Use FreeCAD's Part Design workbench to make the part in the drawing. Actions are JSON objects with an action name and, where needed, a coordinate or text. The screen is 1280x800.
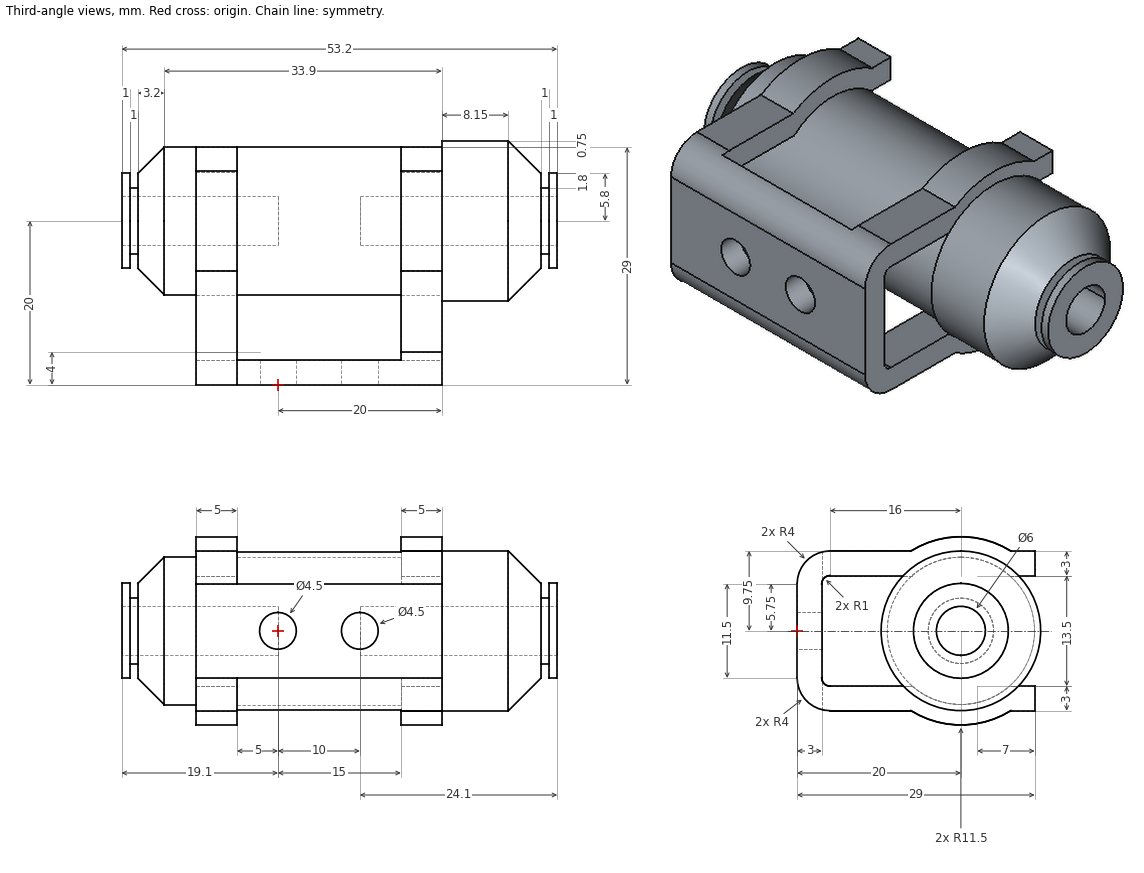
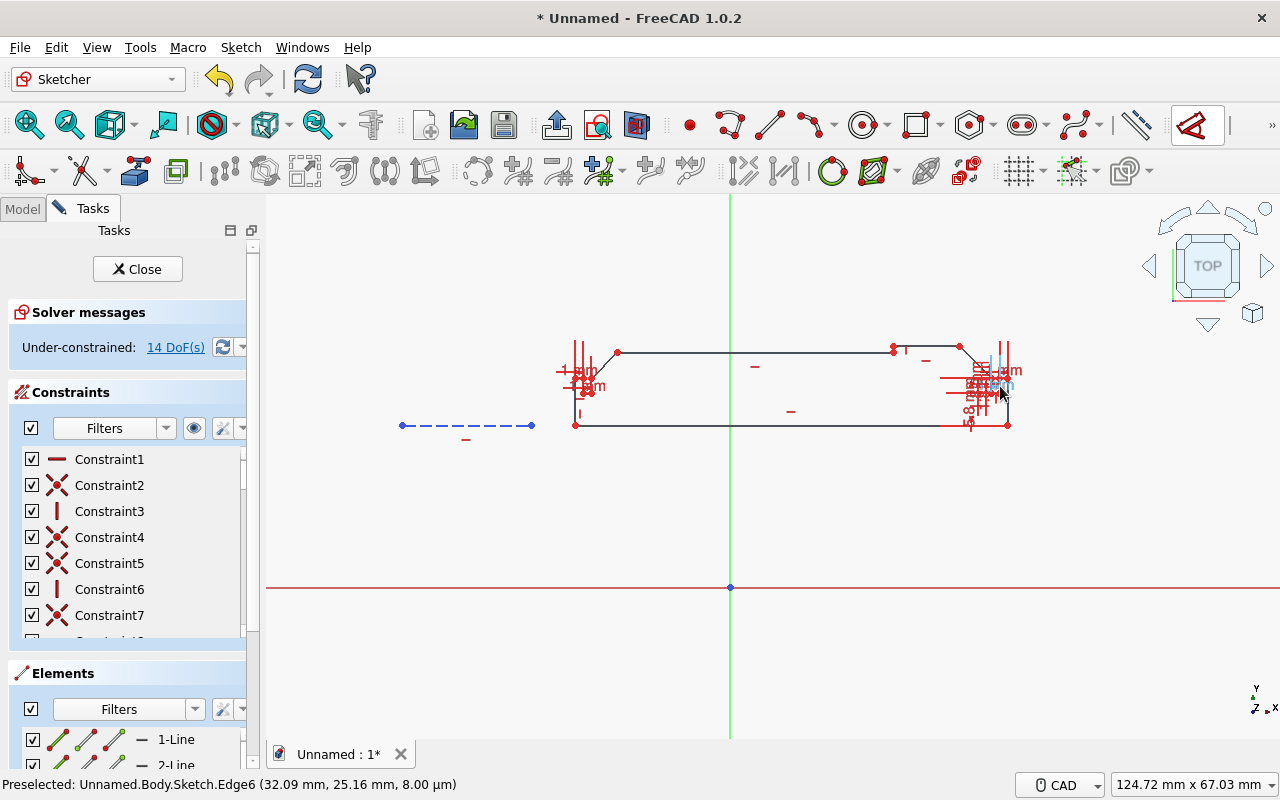
{"action": "scroll", "coordinate": [591, 384], "scroll_direction": "up", "scroll_amount": 6}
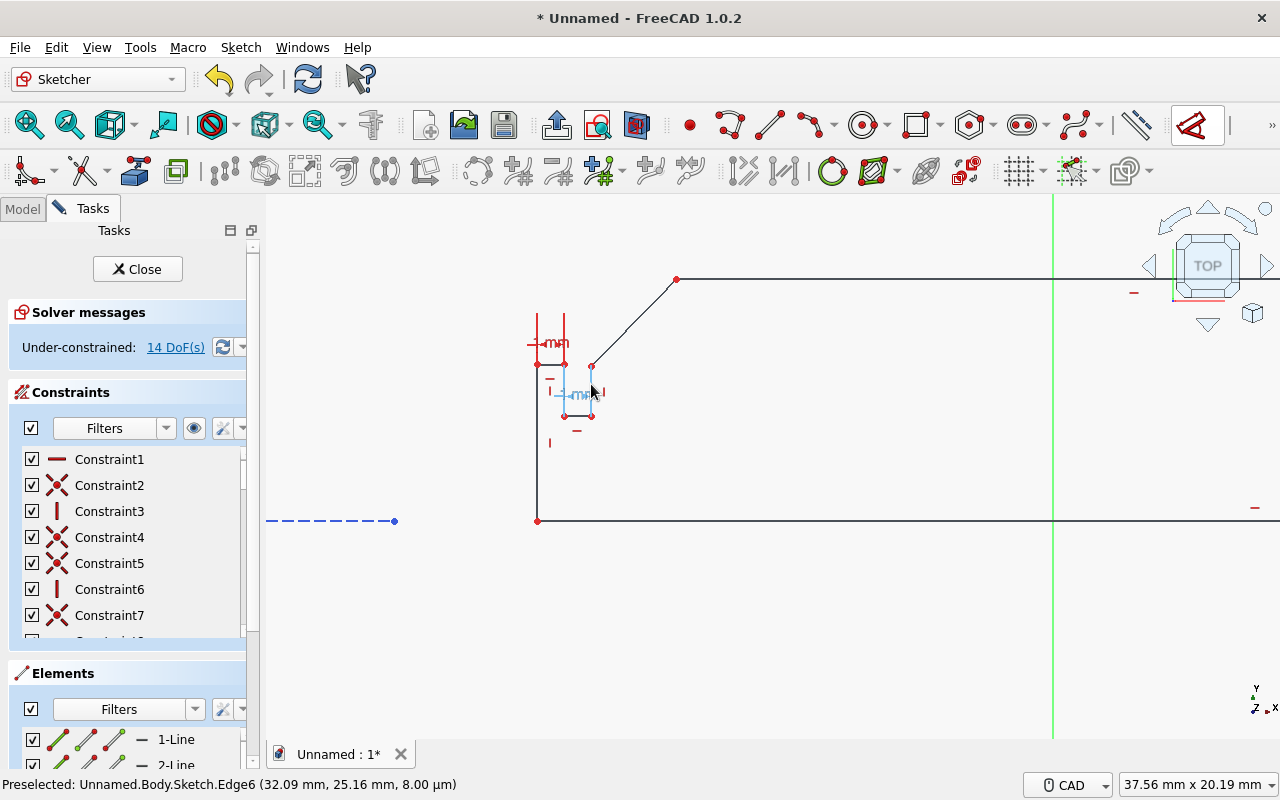
{"action": "left_click", "coordinate": [591, 382]}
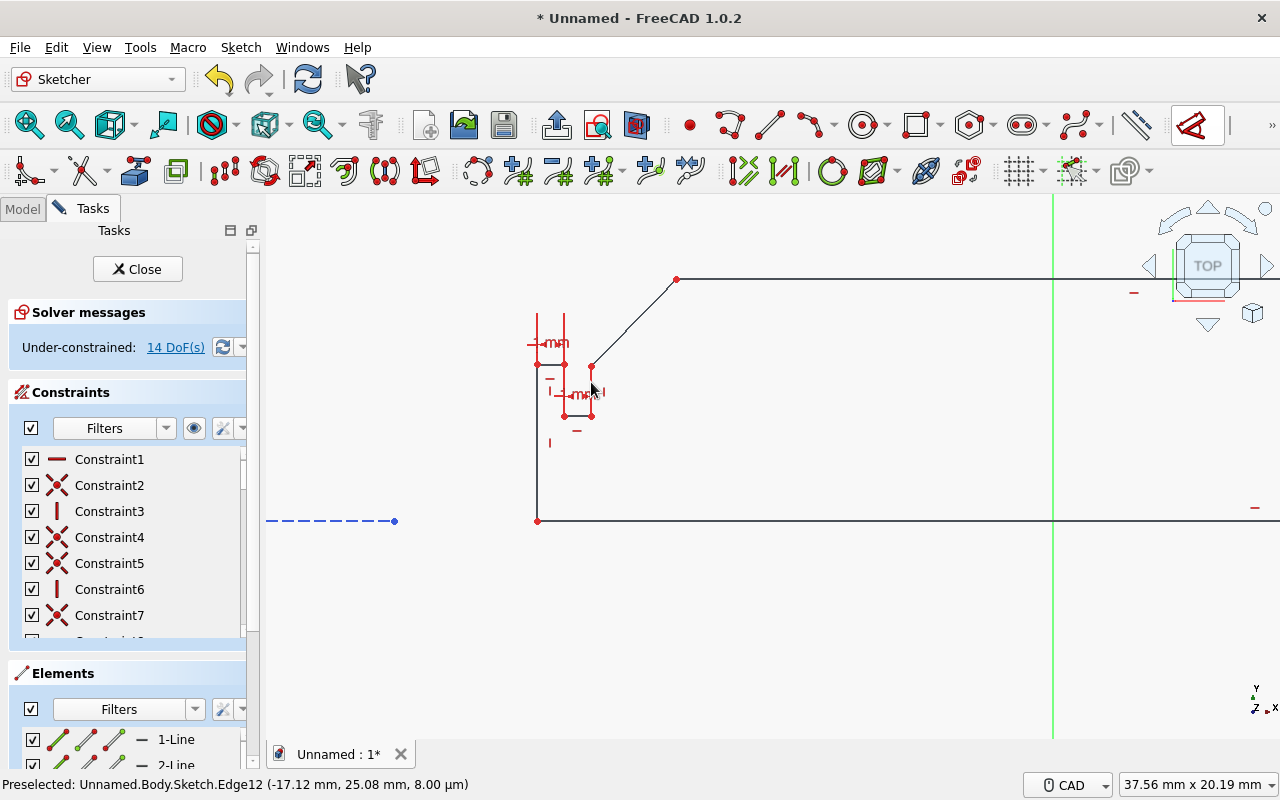
{"action": "left_click", "coordinate": [1218, 126]}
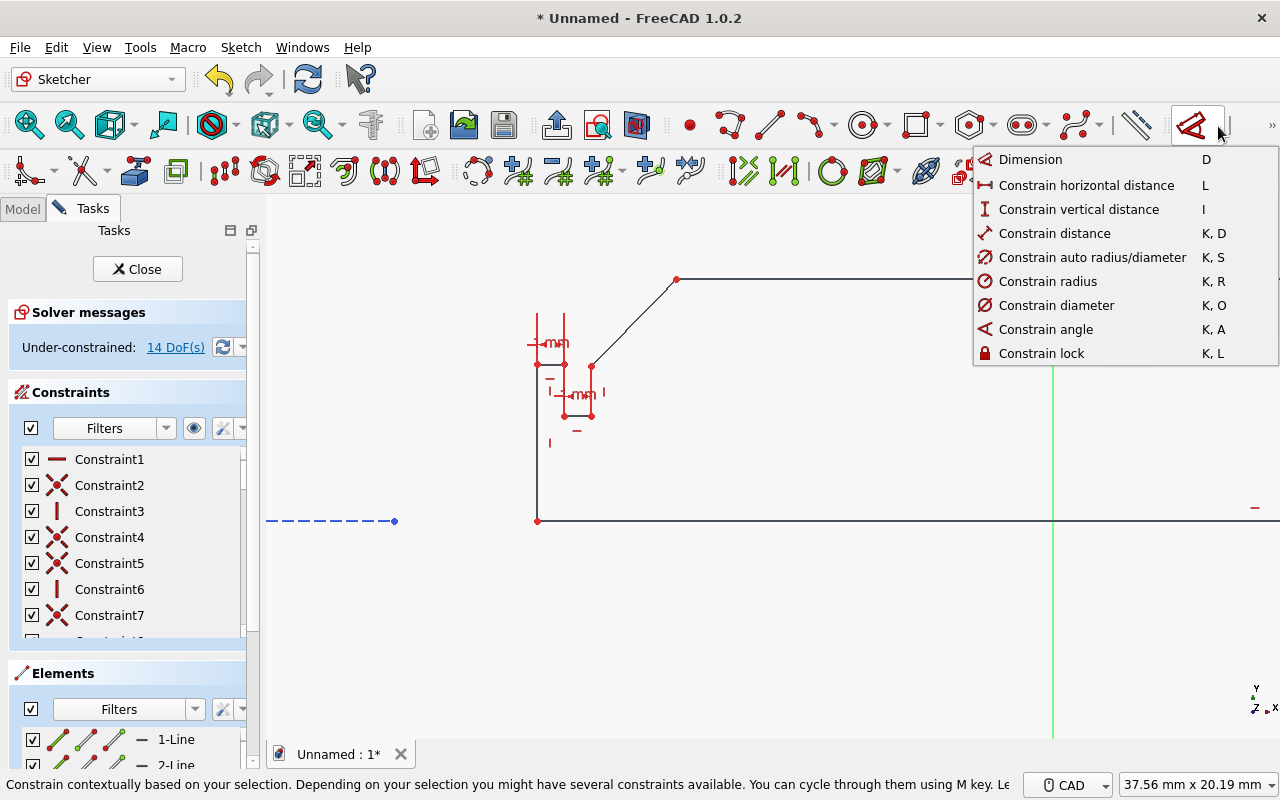
{"action": "left_click", "coordinate": [1126, 209]}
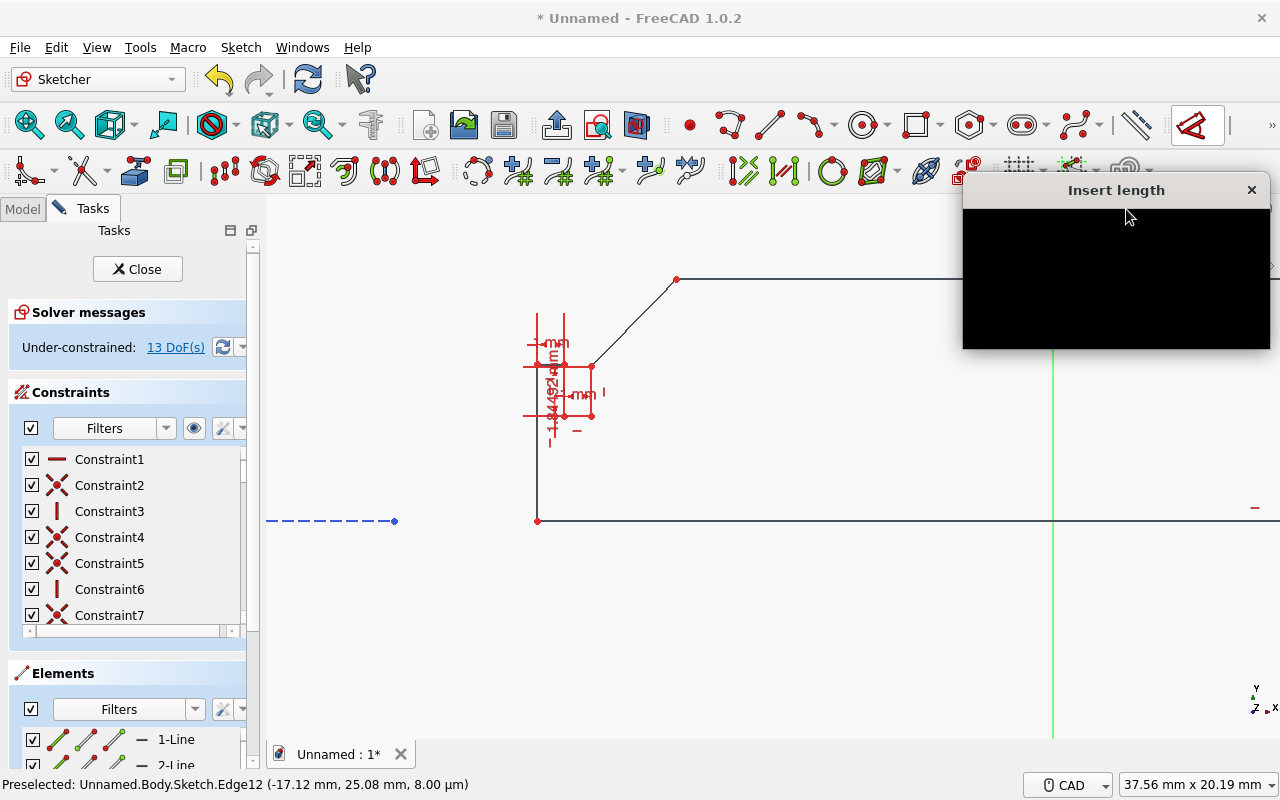
{"action": "type", "text": "1.8"}
{"action": "key", "text": "Return"}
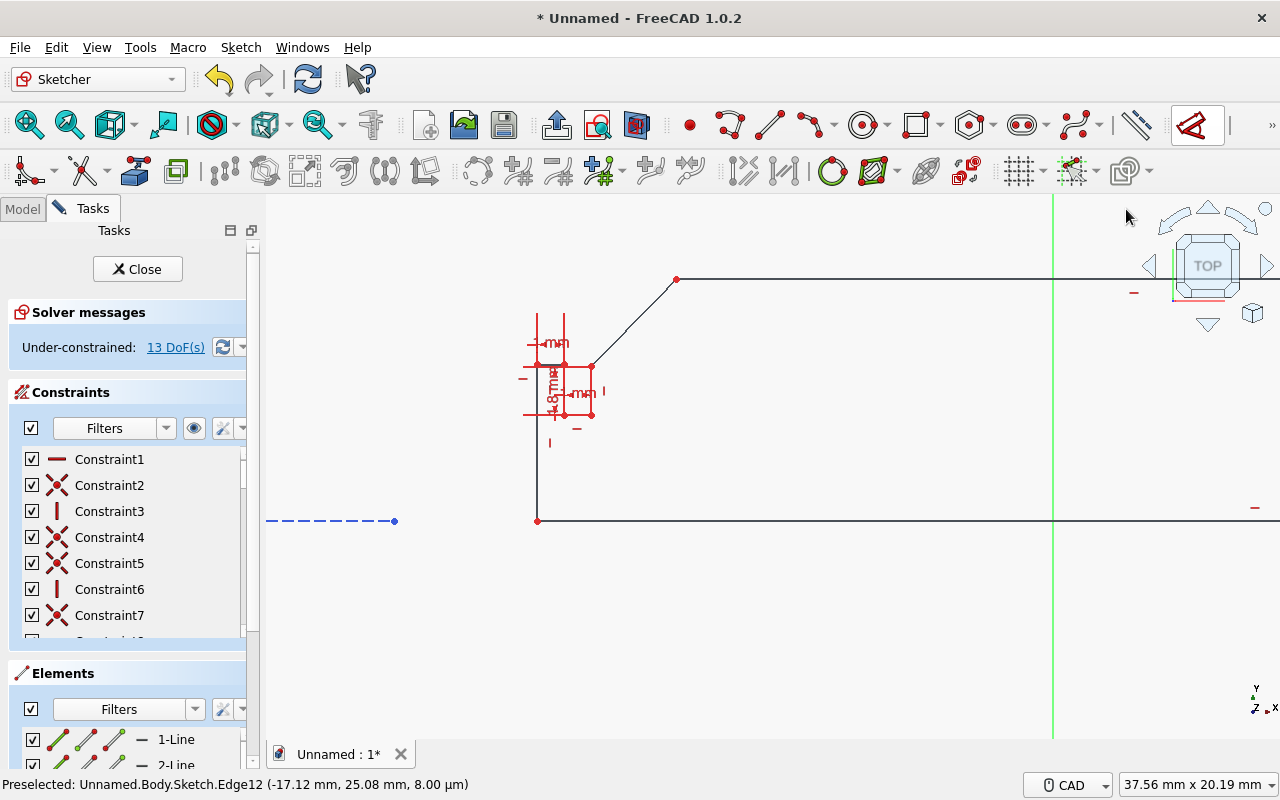
{"action": "left_click", "coordinate": [564, 380]}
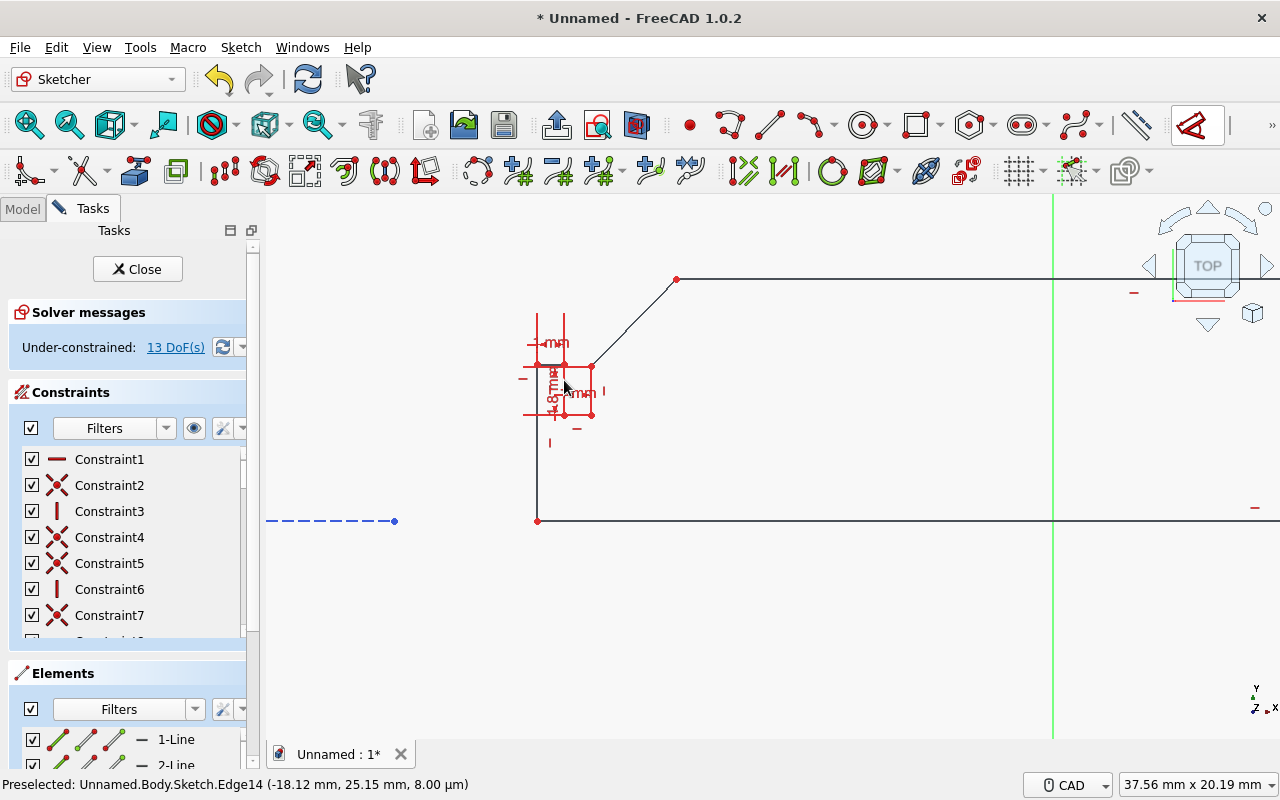
{"action": "left_click", "coordinate": [1218, 126]}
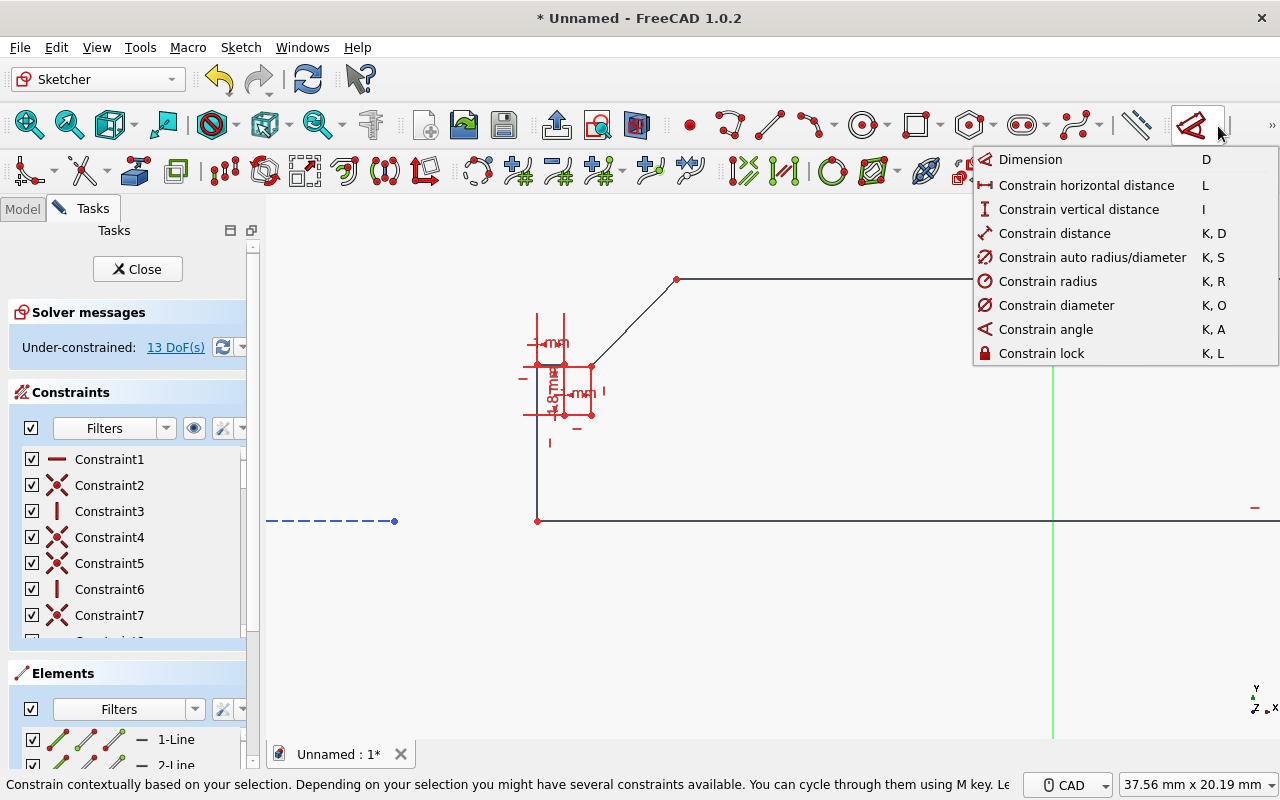
{"action": "left_click", "coordinate": [1126, 209]}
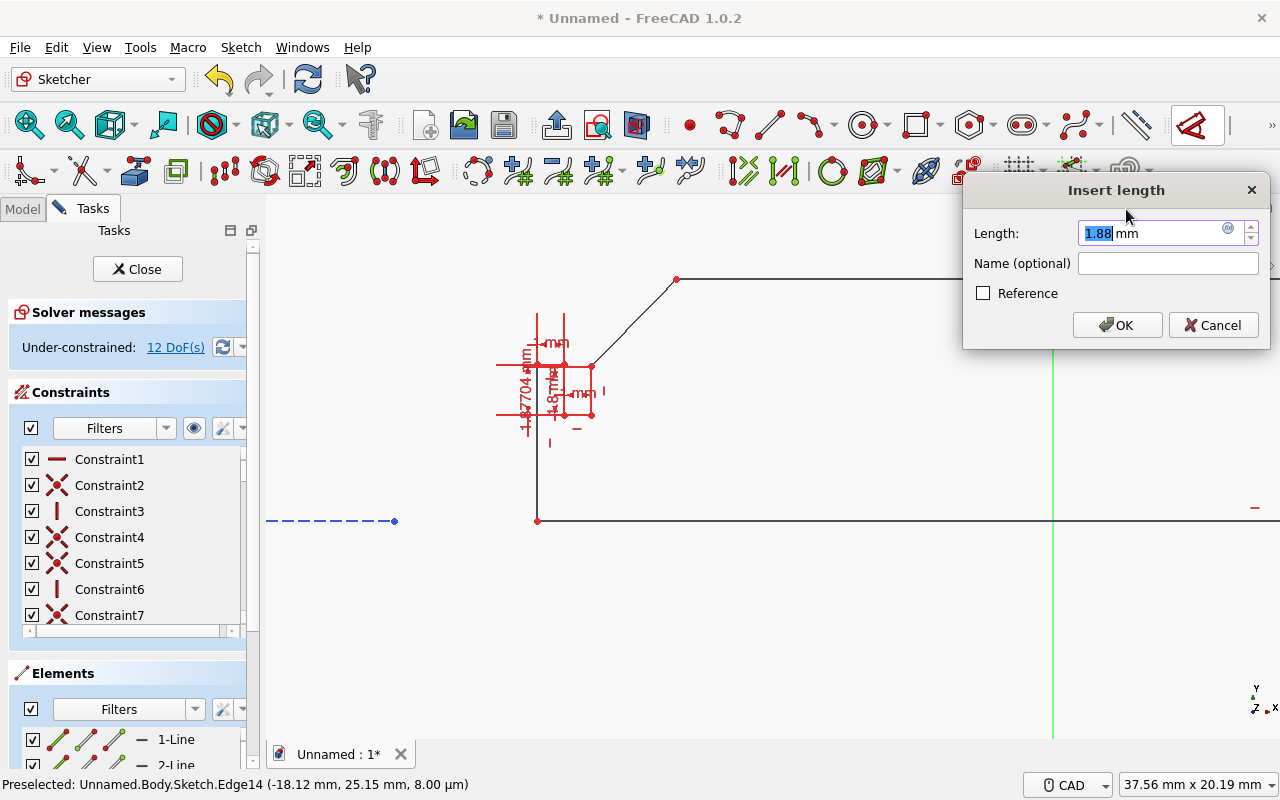
{"action": "type", "text": "1.8"}
{"action": "key", "text": "Return"}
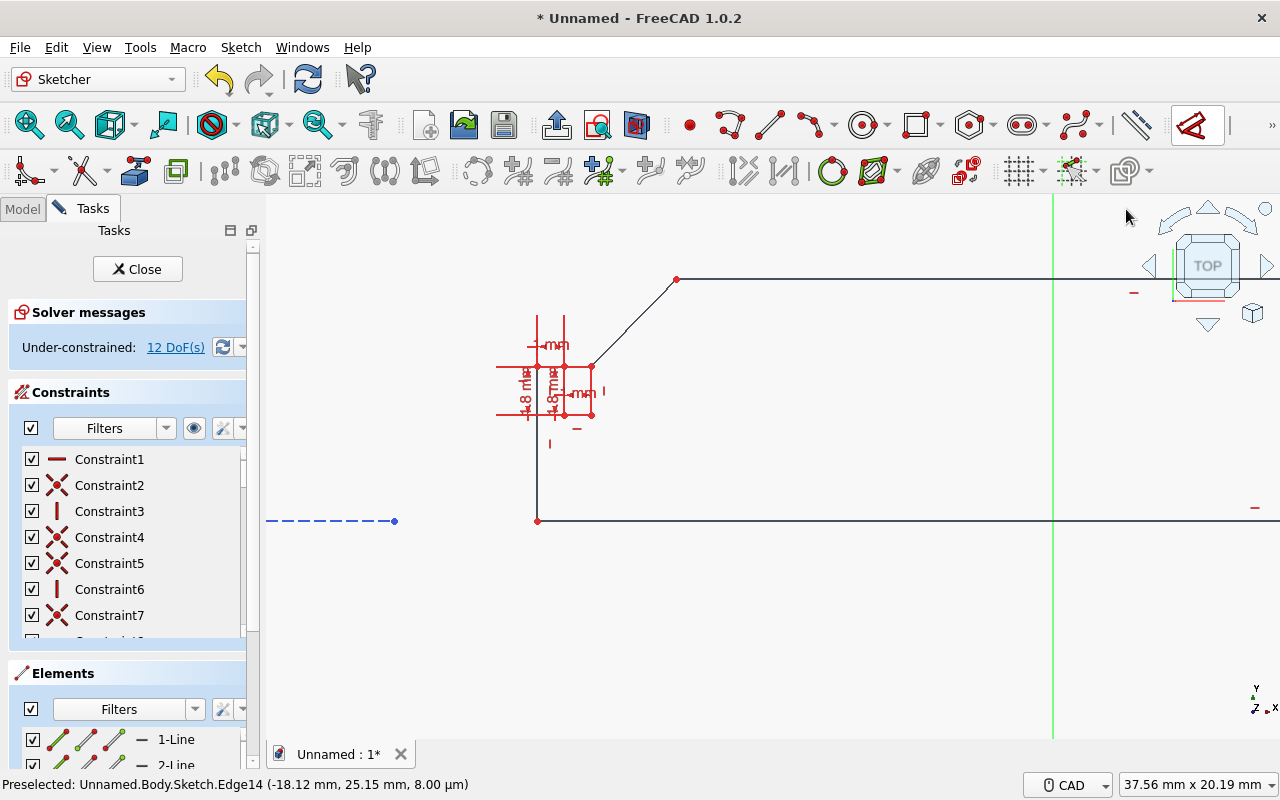
{"action": "left_click", "coordinate": [537, 413]}